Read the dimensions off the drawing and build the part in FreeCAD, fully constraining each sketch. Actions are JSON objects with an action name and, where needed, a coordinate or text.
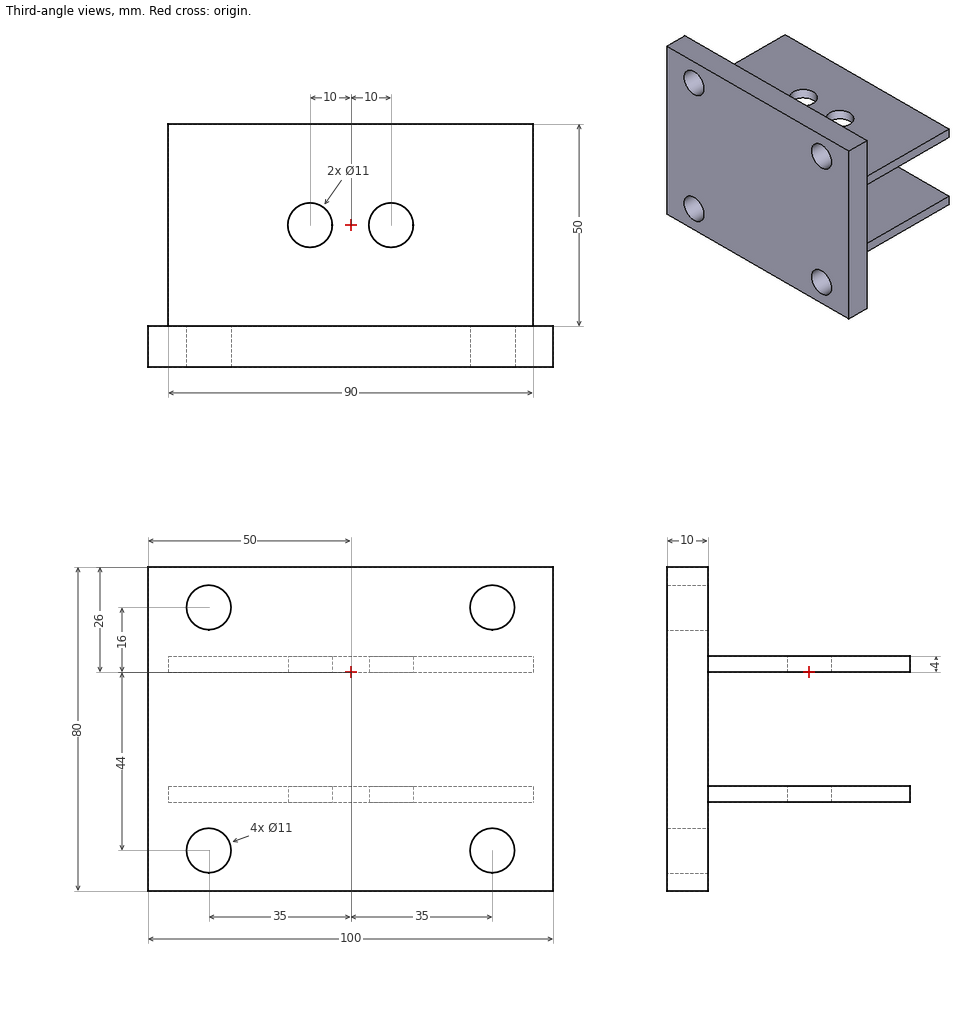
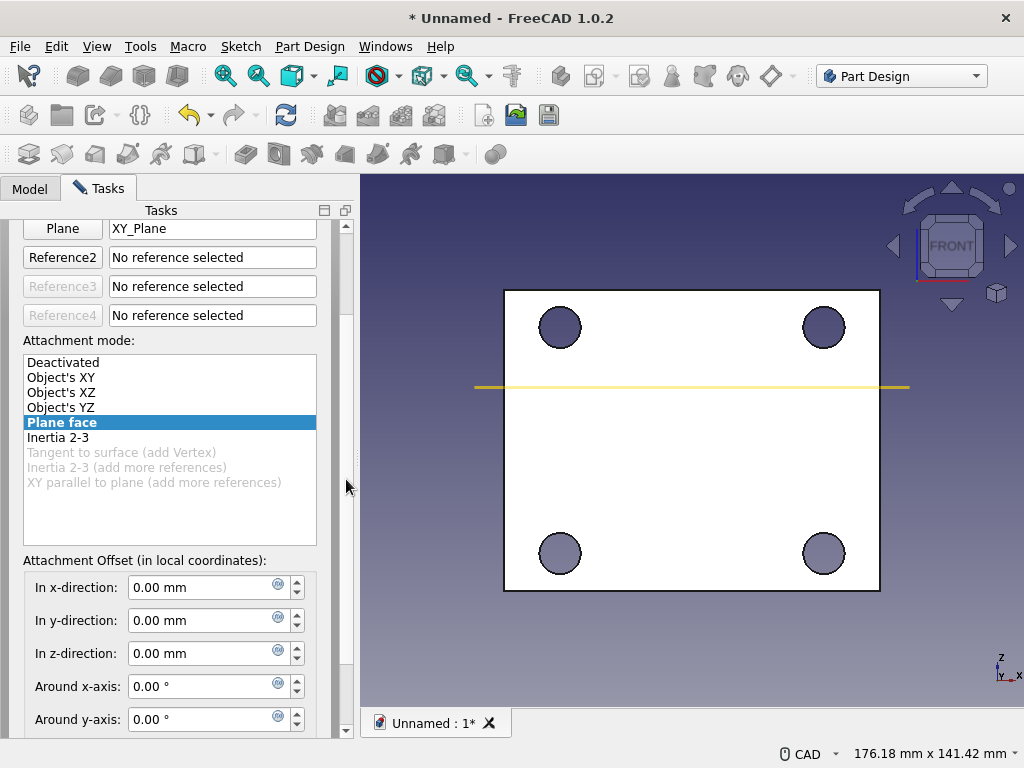
{"action": "triple_click", "coordinate": [210, 654]}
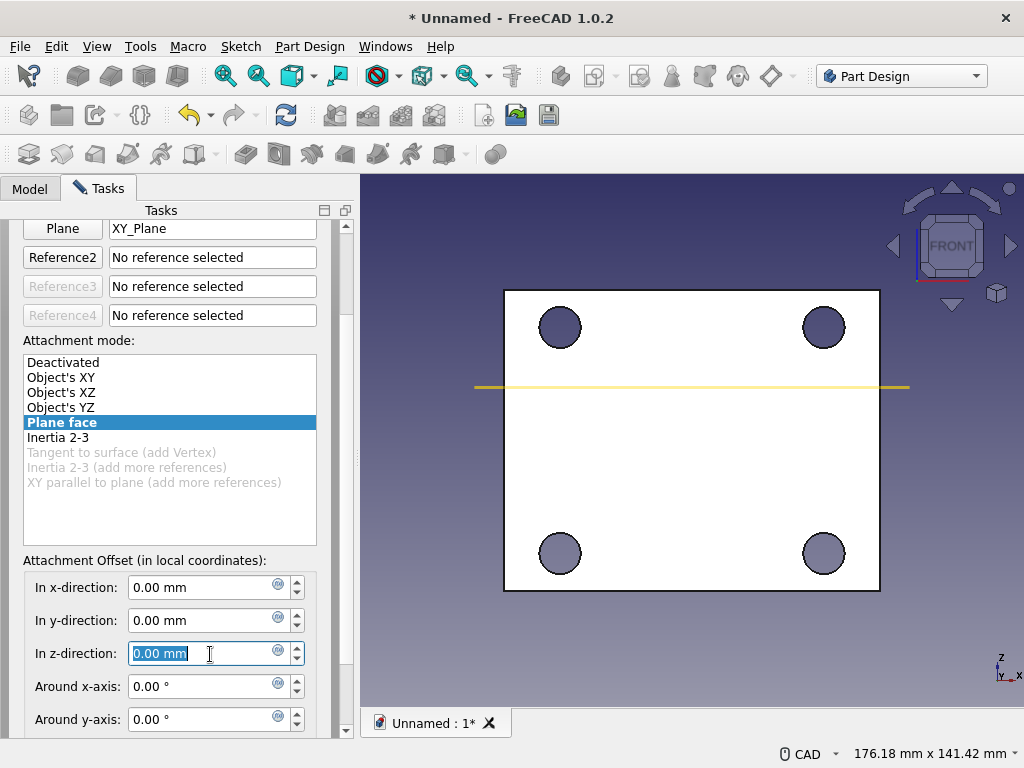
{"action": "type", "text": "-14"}
{"action": "key", "text": "Tab"}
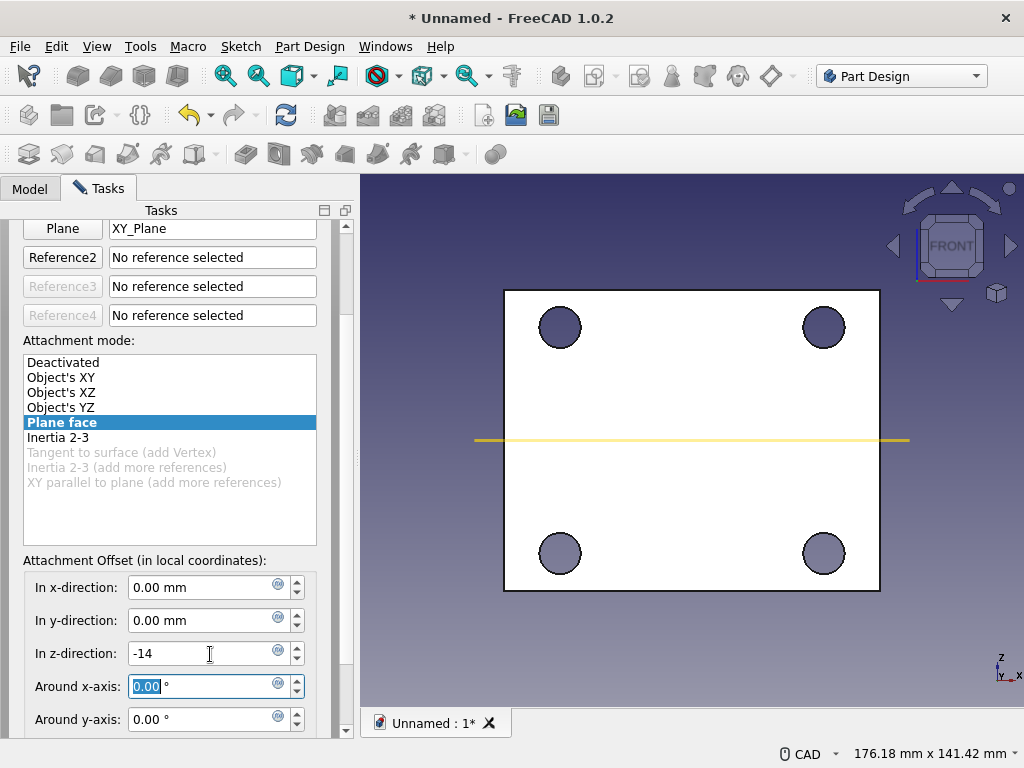
{"action": "scroll", "coordinate": [346, 479], "scroll_direction": "up", "scroll_amount": 3}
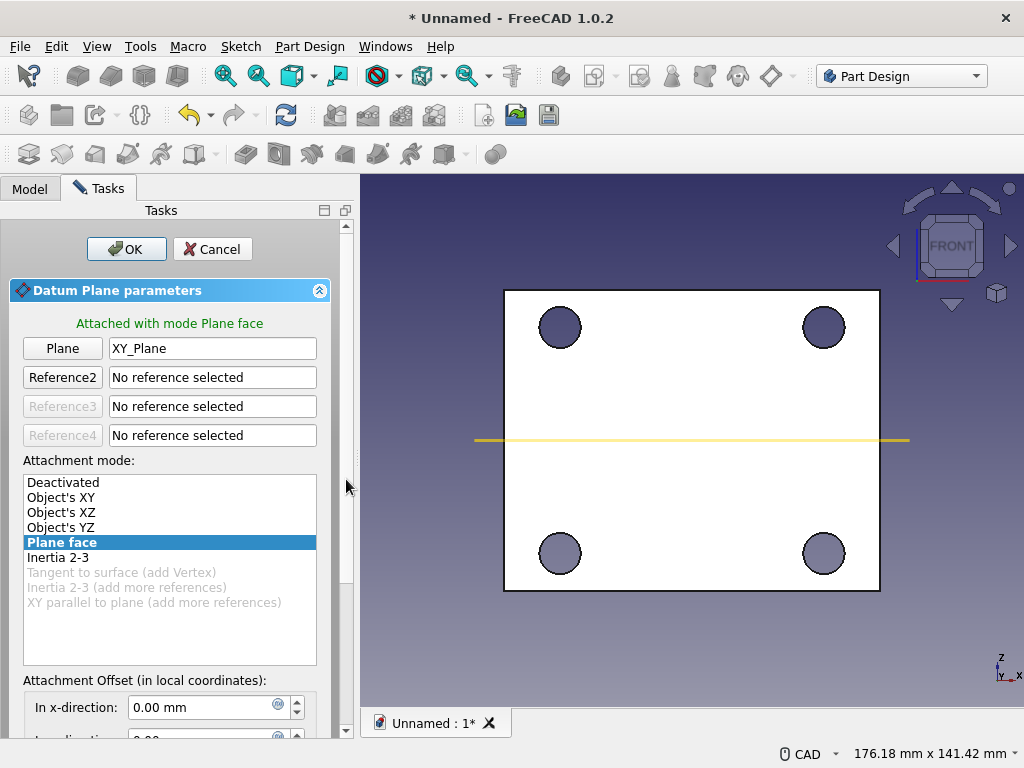
{"action": "left_click", "coordinate": [127, 249]}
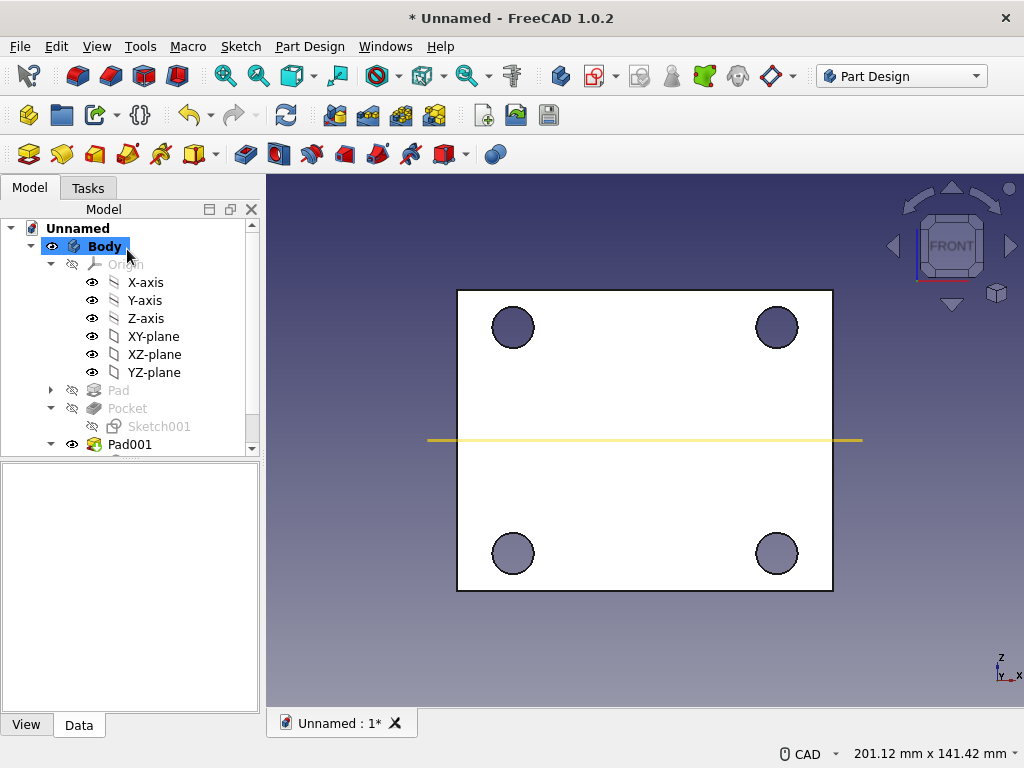
{"action": "left_click", "coordinate": [117, 390]}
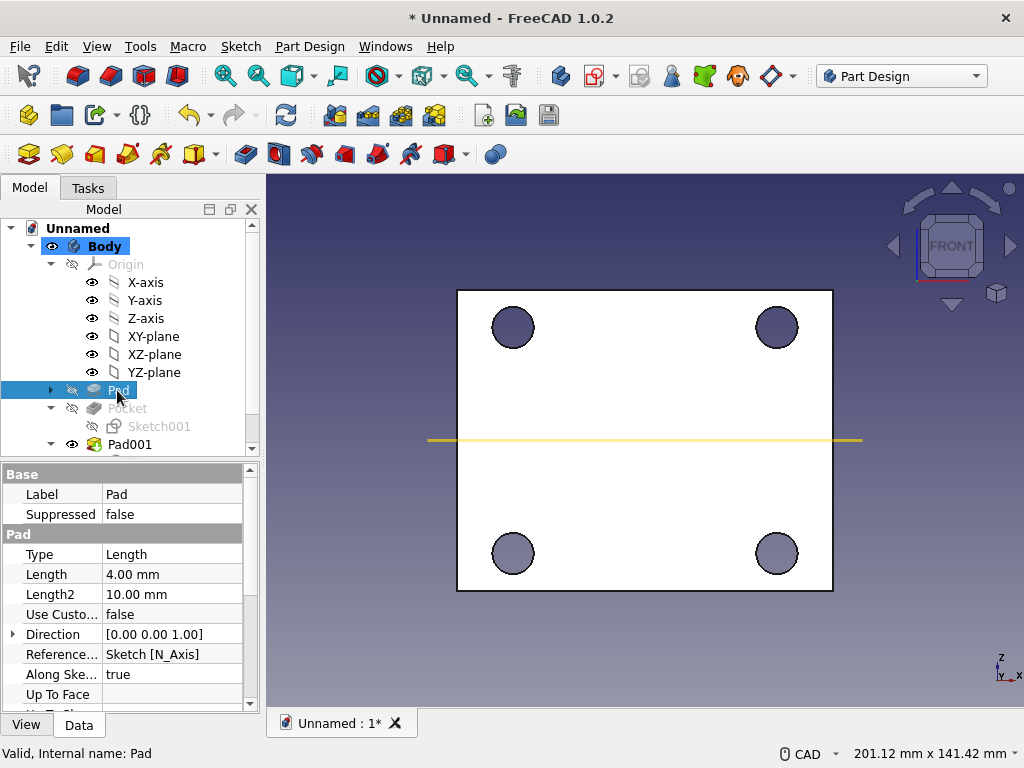
{"action": "left_click", "coordinate": [335, 116]}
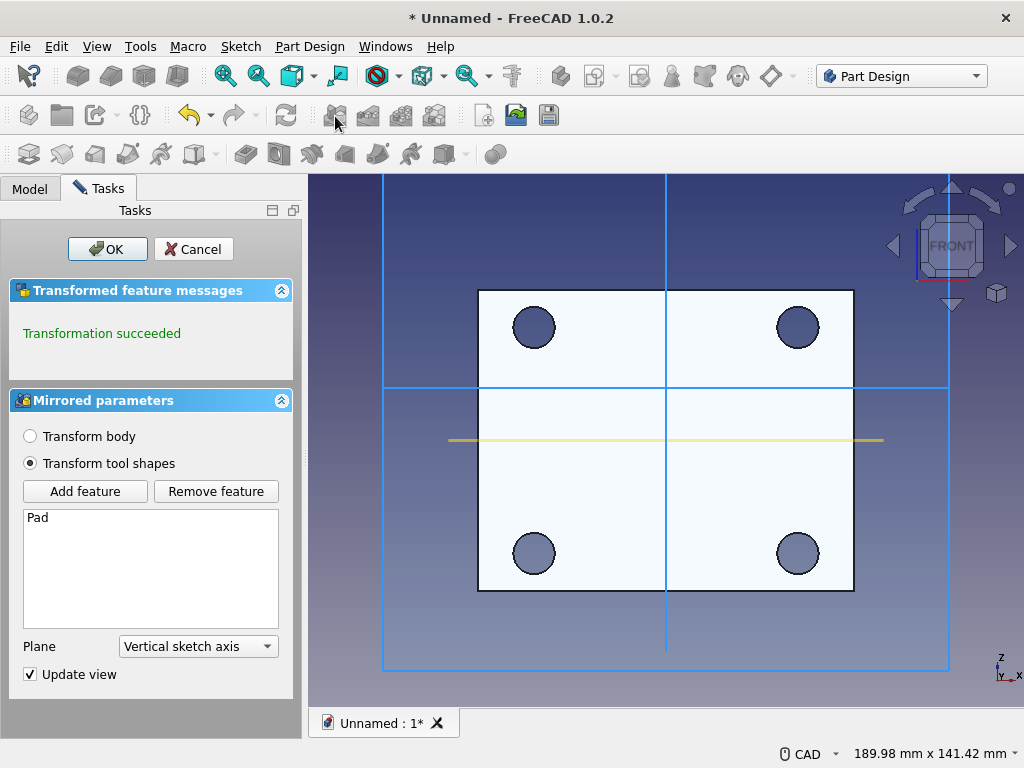
{"action": "left_click", "coordinate": [199, 646]}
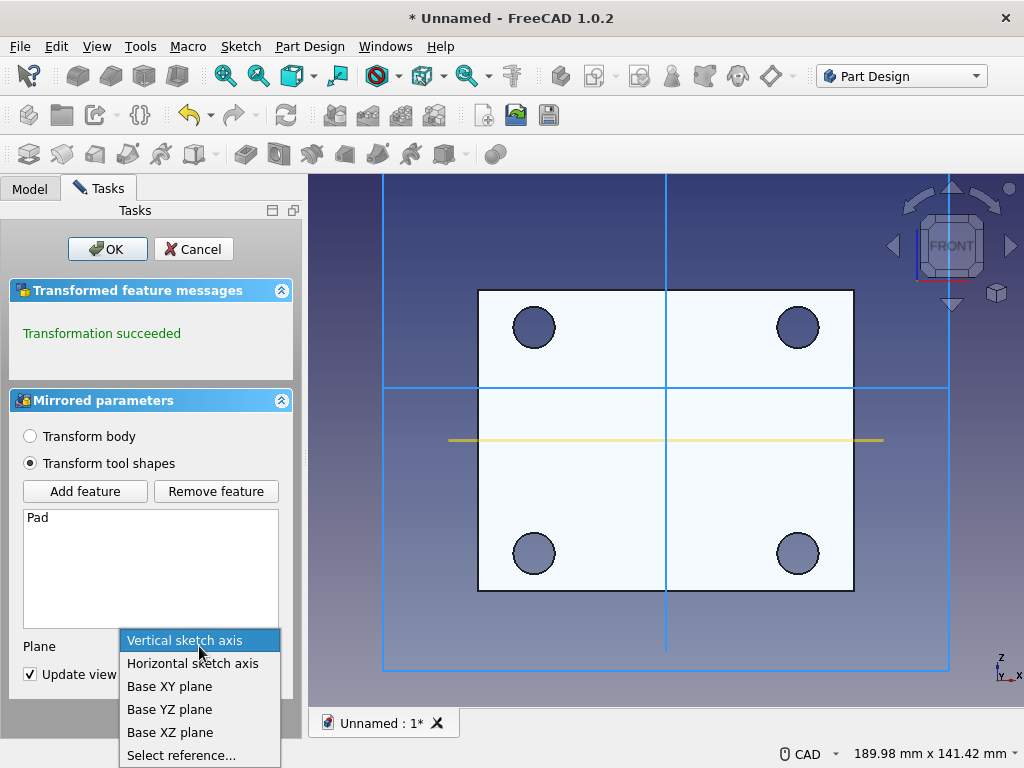
{"action": "left_click", "coordinate": [198, 756]}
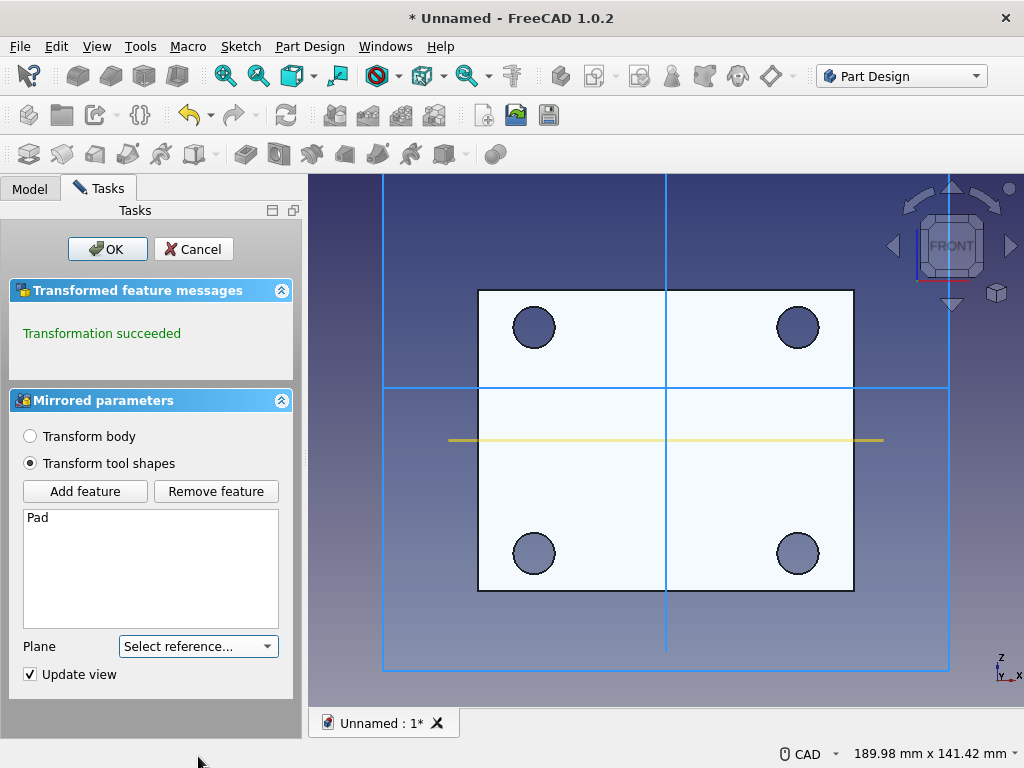
{"action": "left_click", "coordinate": [30, 188]}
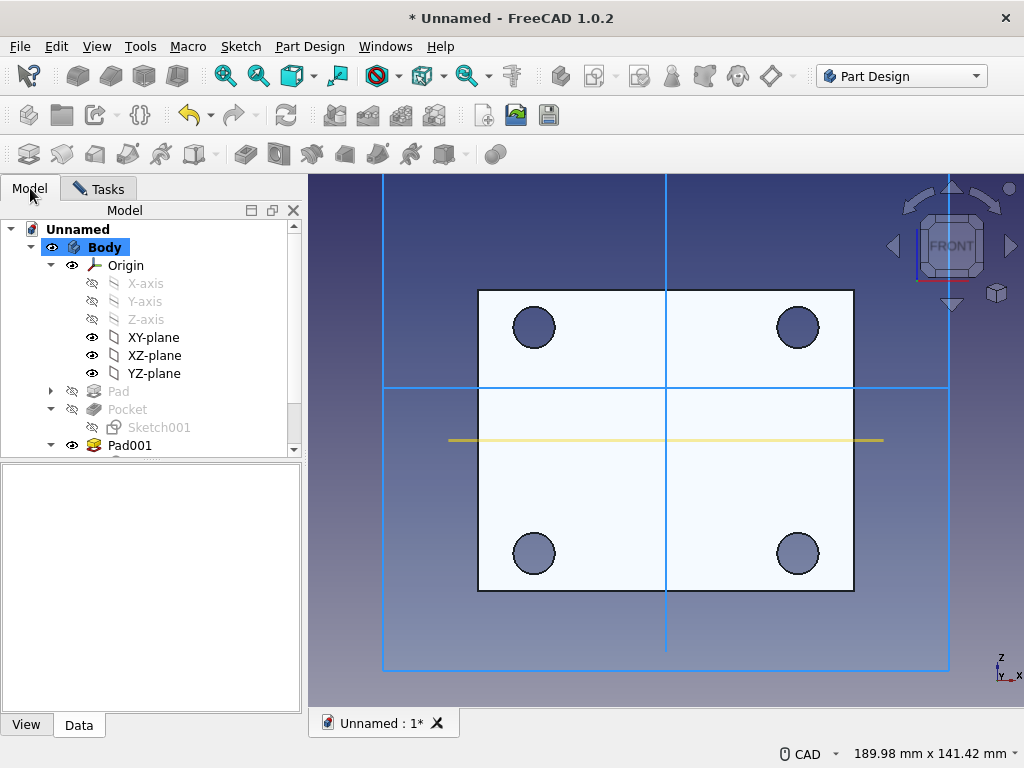
{"action": "scroll", "coordinate": [101, 333], "scroll_direction": "down", "scroll_amount": 3}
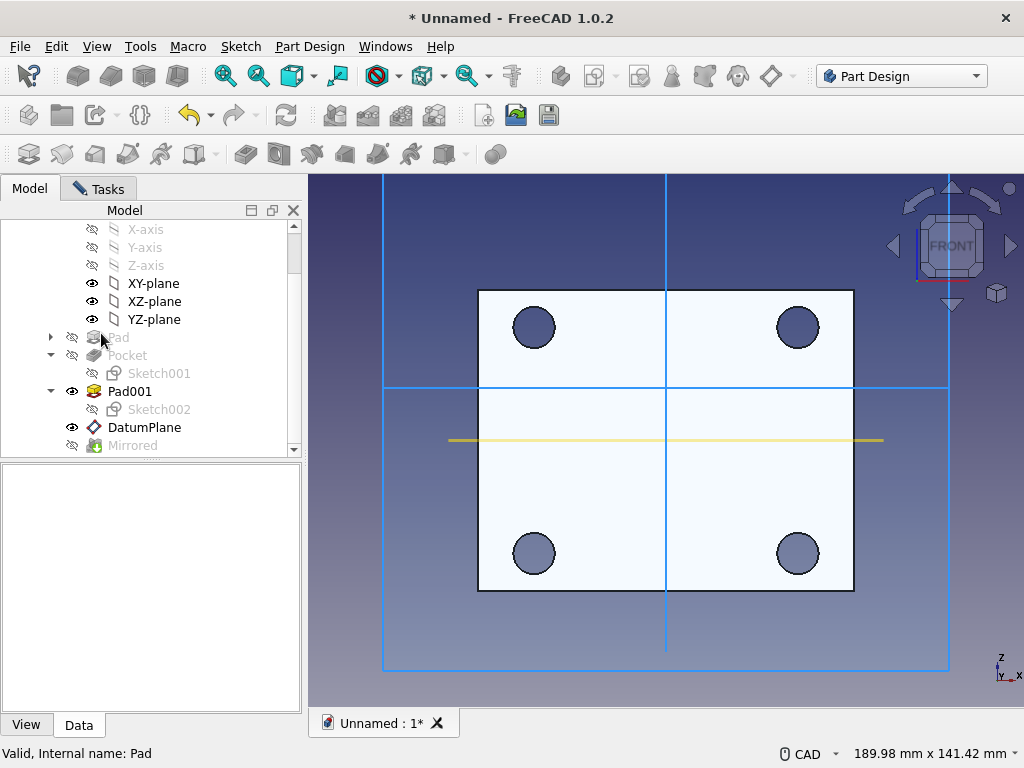
{"action": "left_click", "coordinate": [117, 427]}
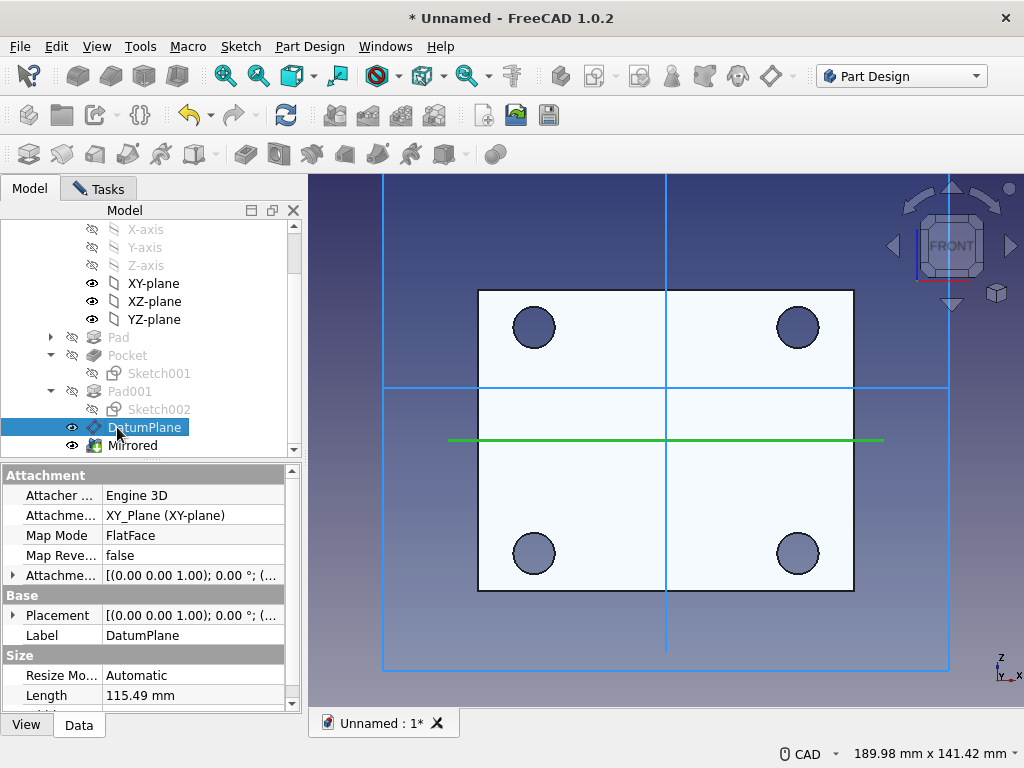
{"action": "left_click", "coordinate": [98, 188]}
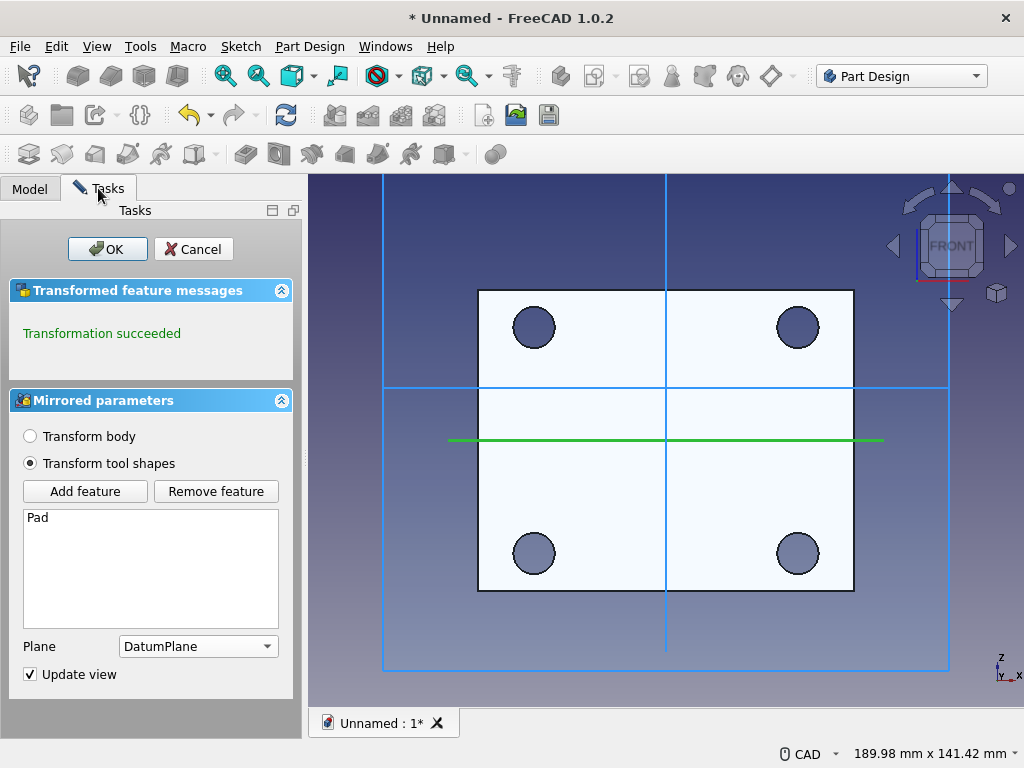
{"action": "left_click", "coordinate": [108, 249]}